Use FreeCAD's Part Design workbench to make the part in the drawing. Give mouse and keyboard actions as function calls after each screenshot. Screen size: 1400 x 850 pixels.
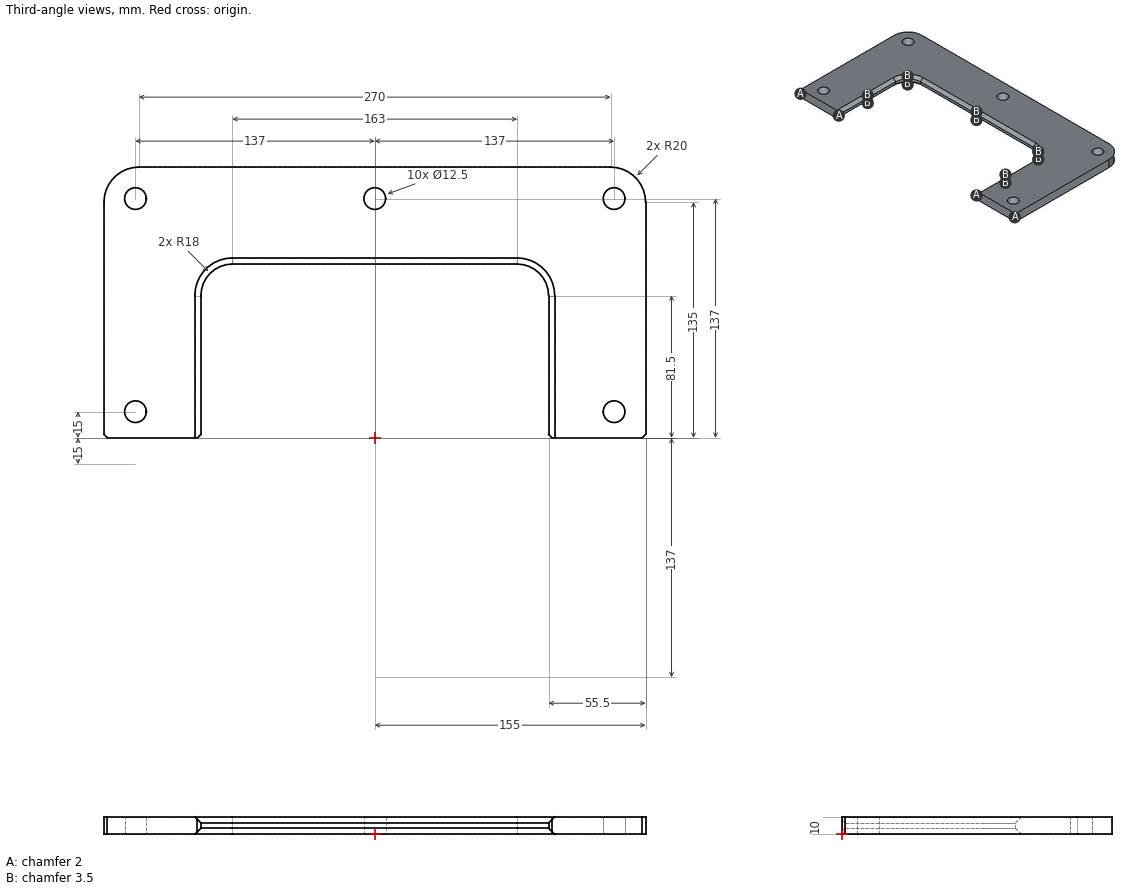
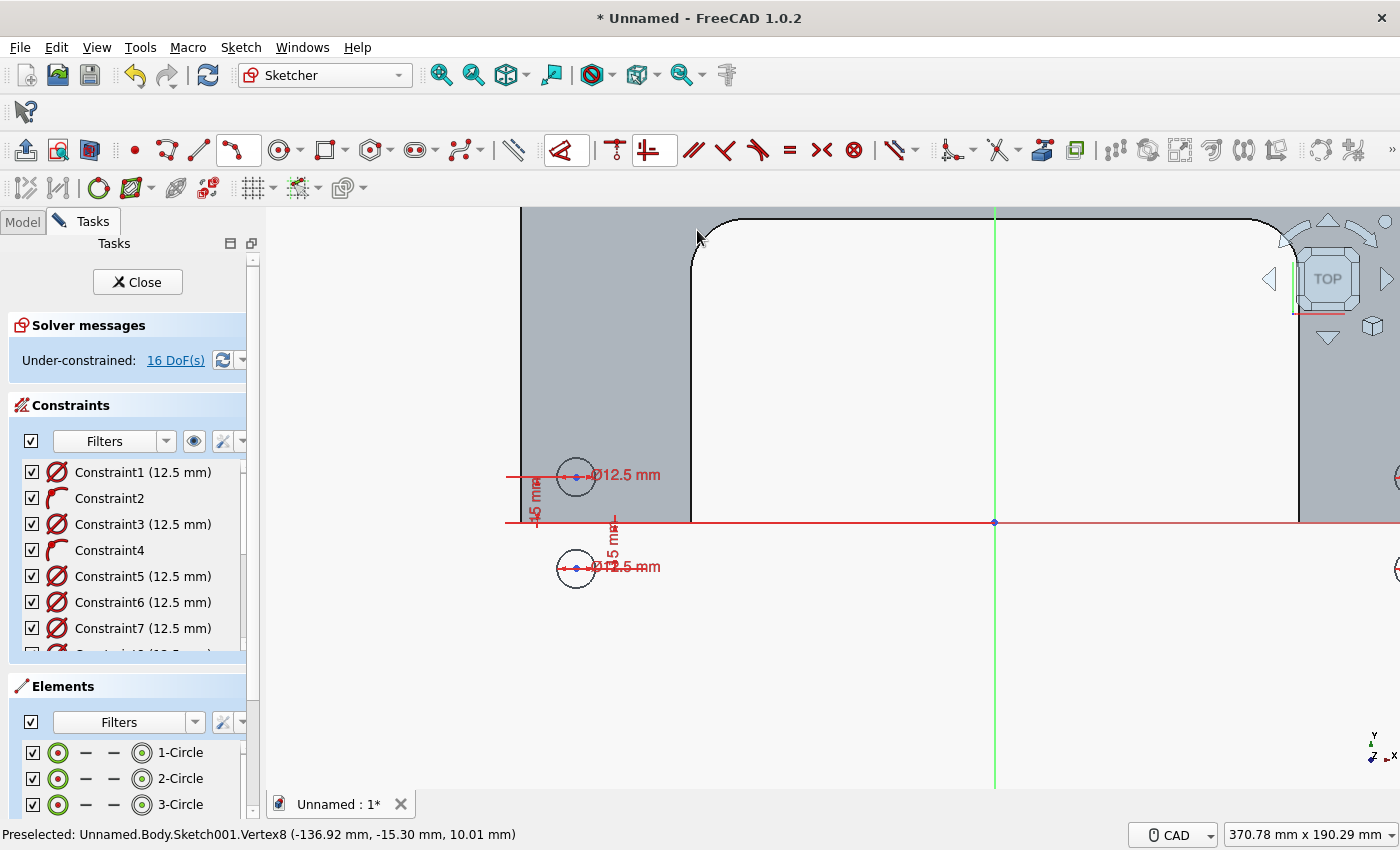
scroll(576, 478, down, 4)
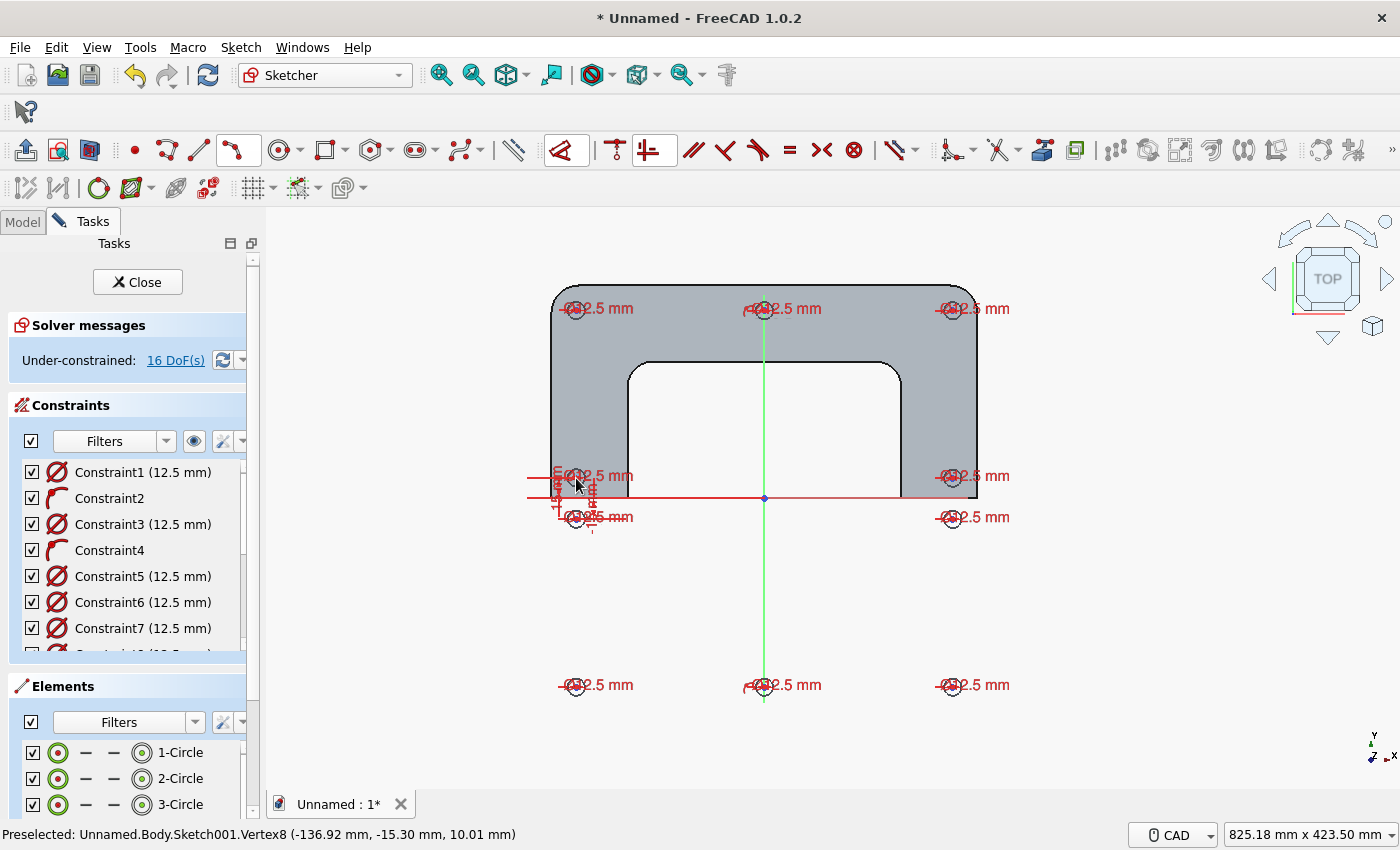
scroll(953, 519, up, 4)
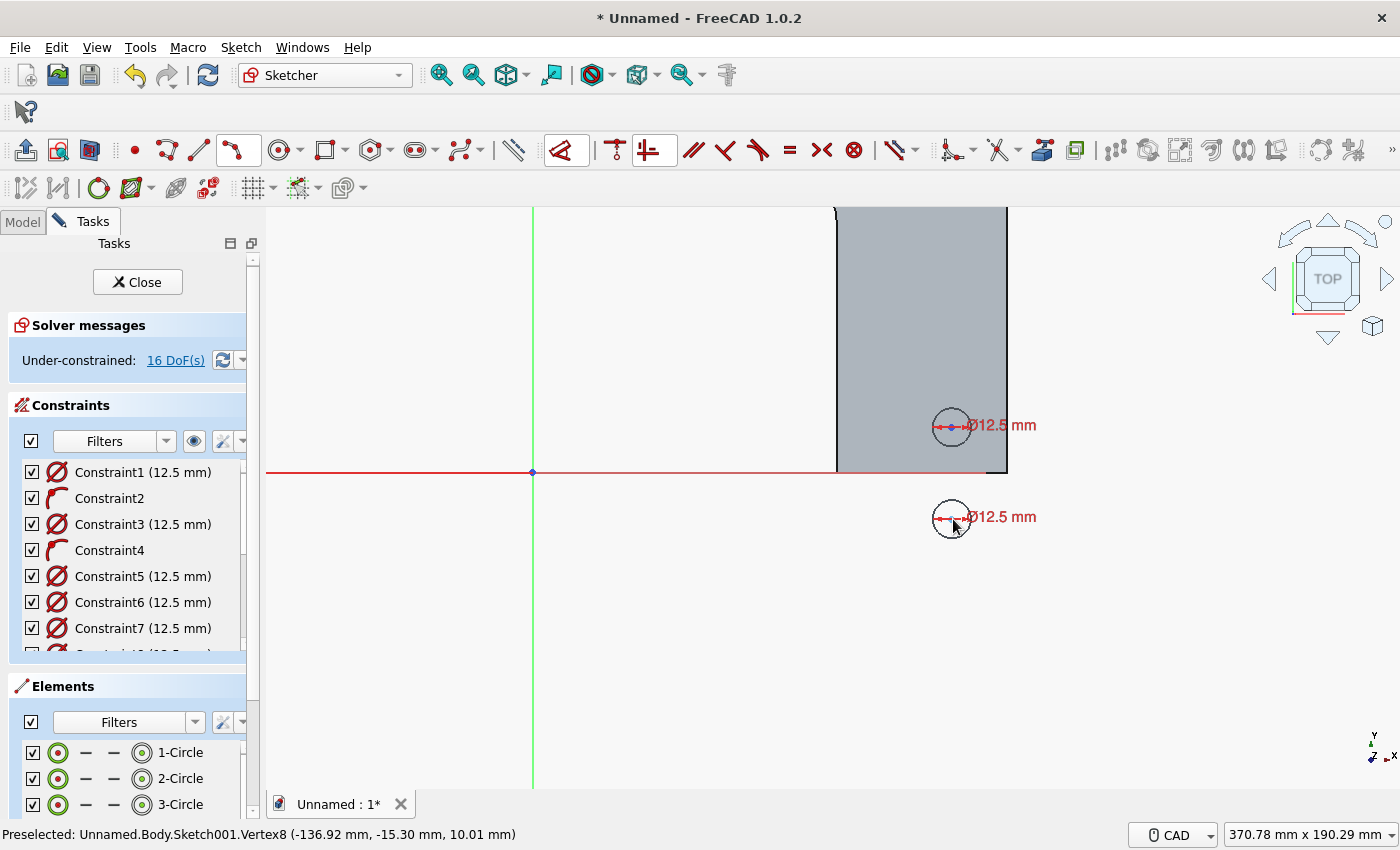
click(952, 519)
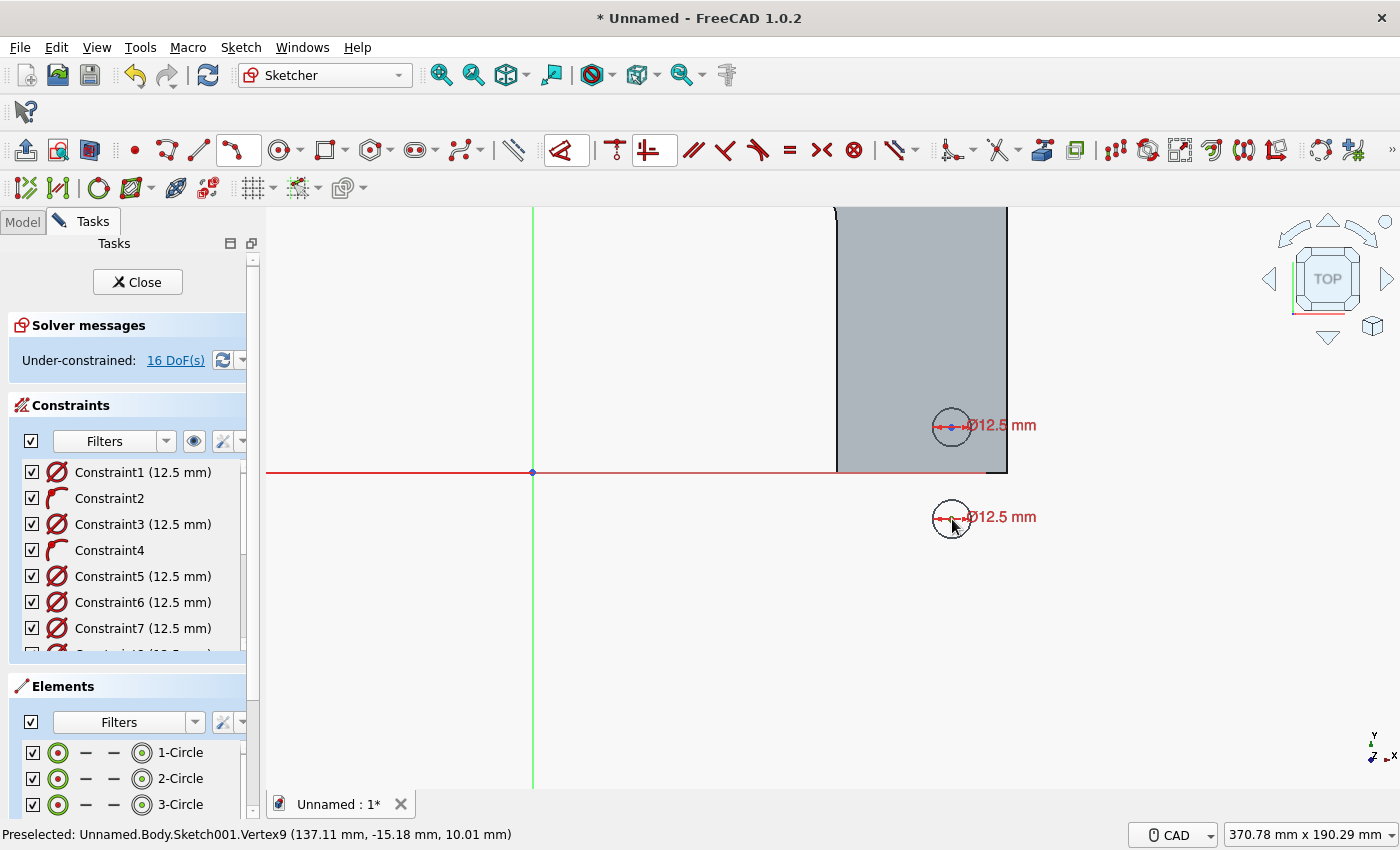
click(584, 150)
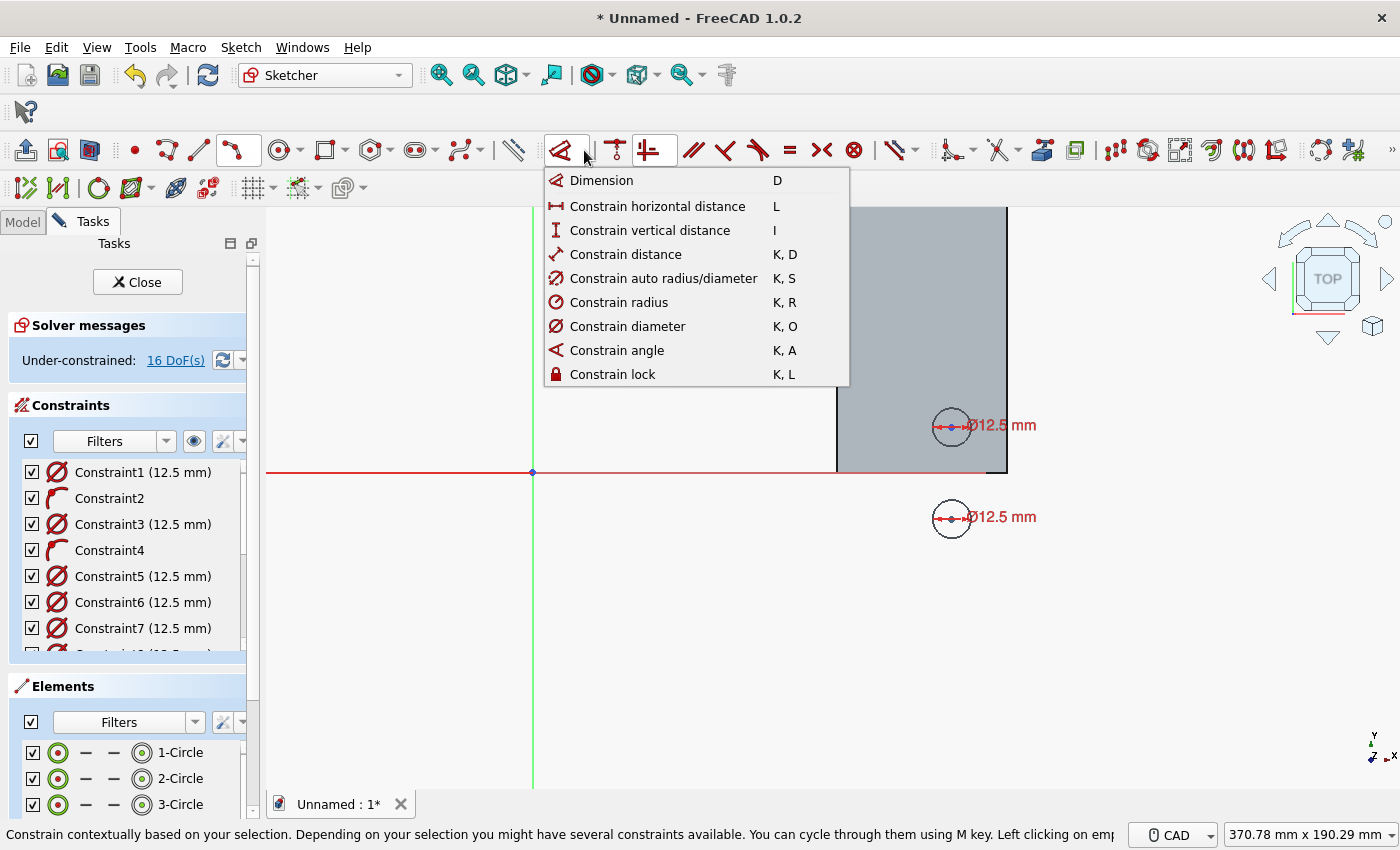
click(697, 230)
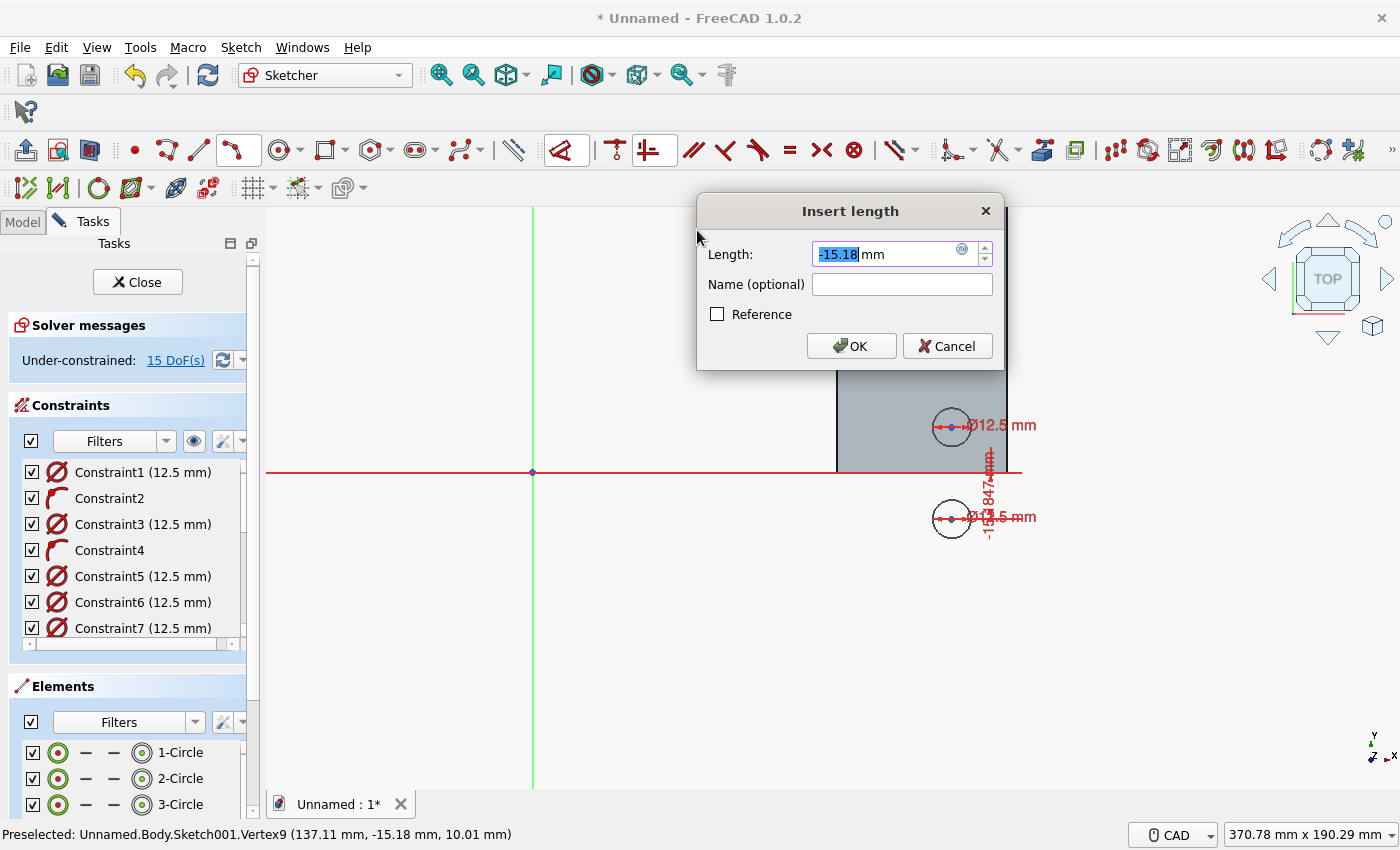
text(-15)
key(Return)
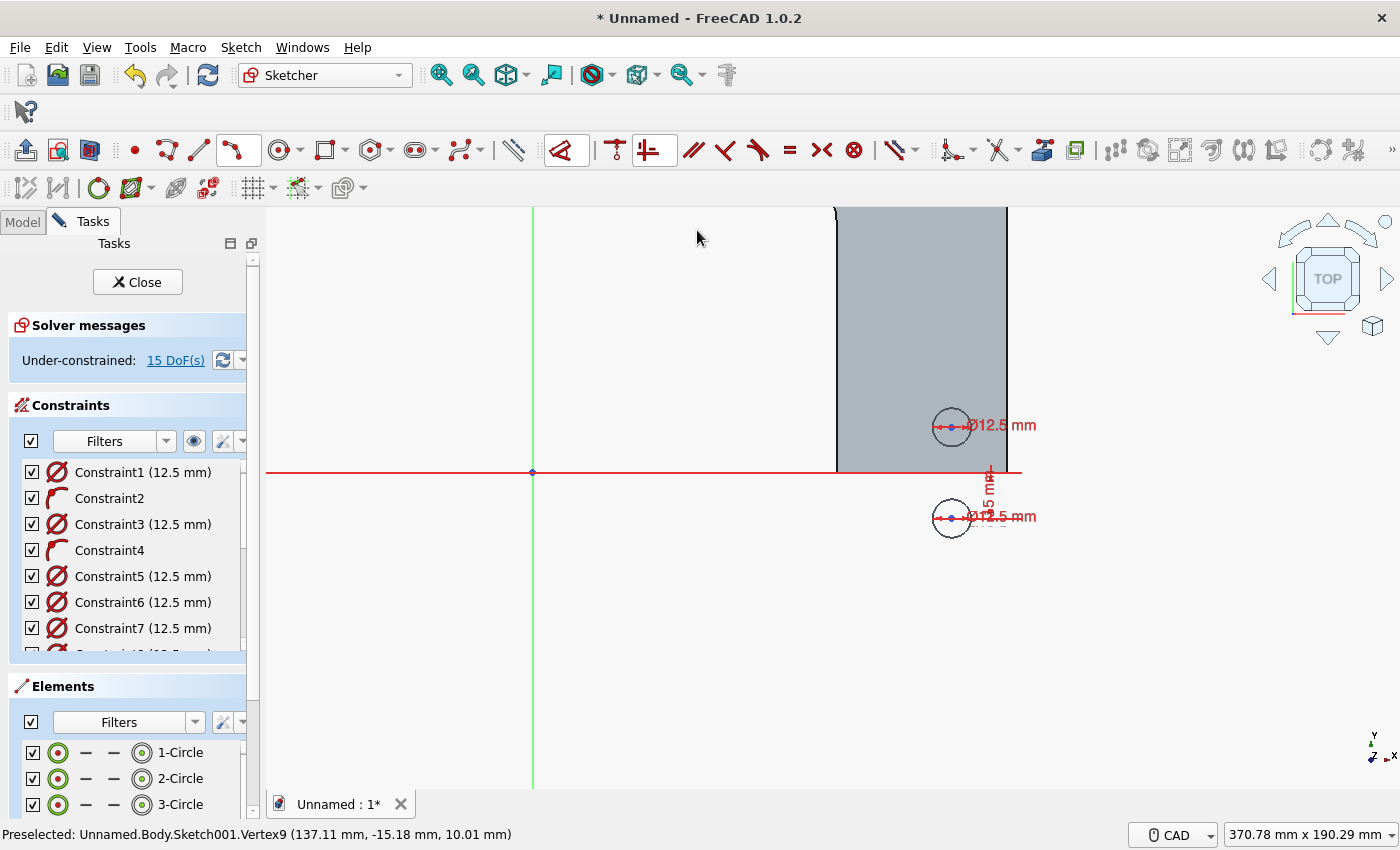
click(952, 427)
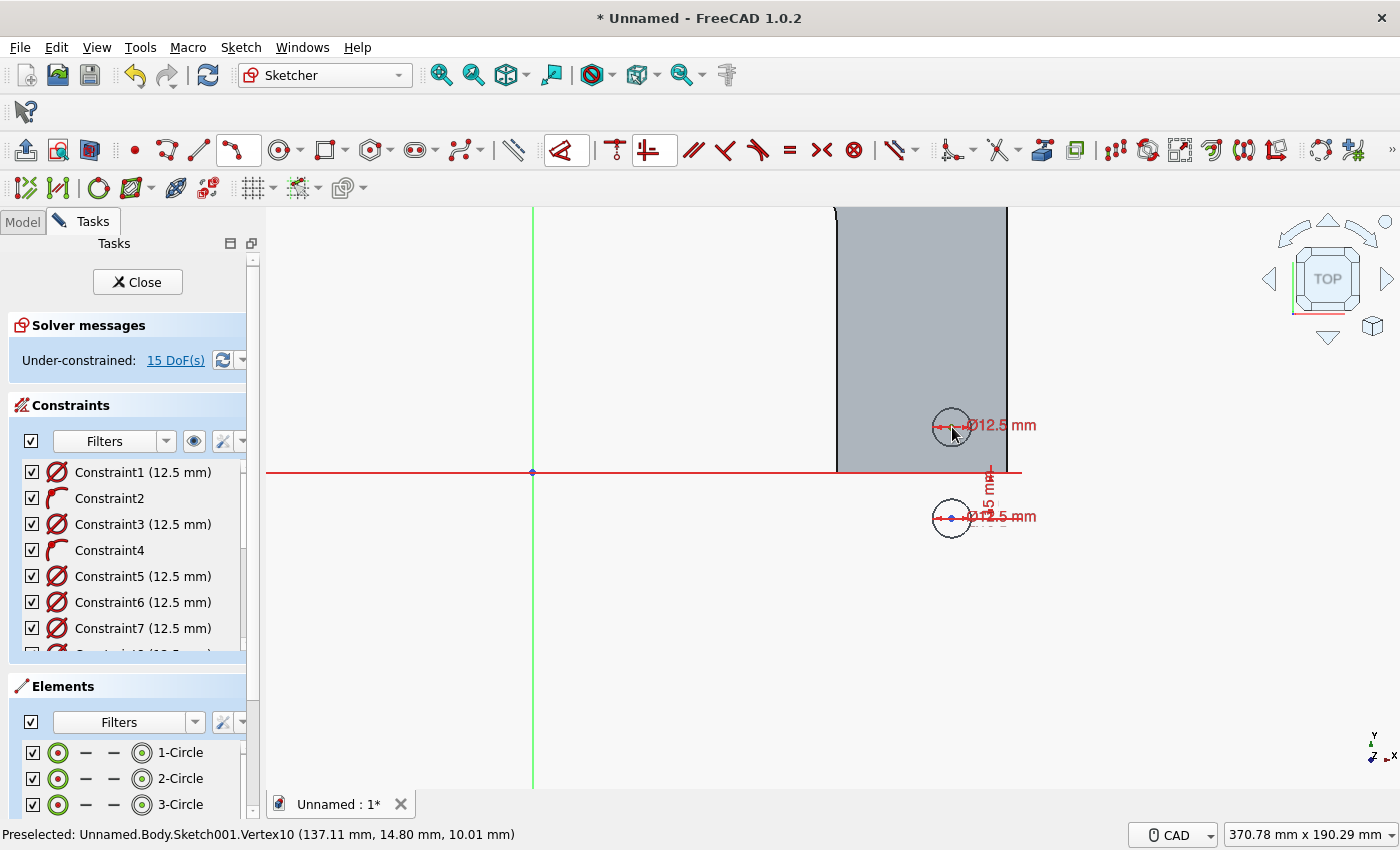
key(i)